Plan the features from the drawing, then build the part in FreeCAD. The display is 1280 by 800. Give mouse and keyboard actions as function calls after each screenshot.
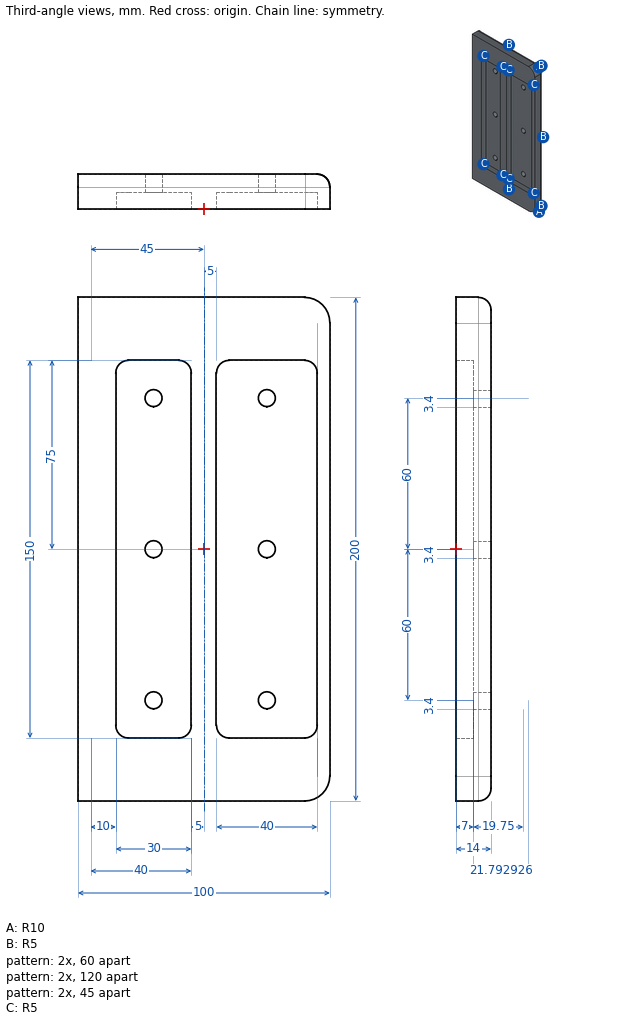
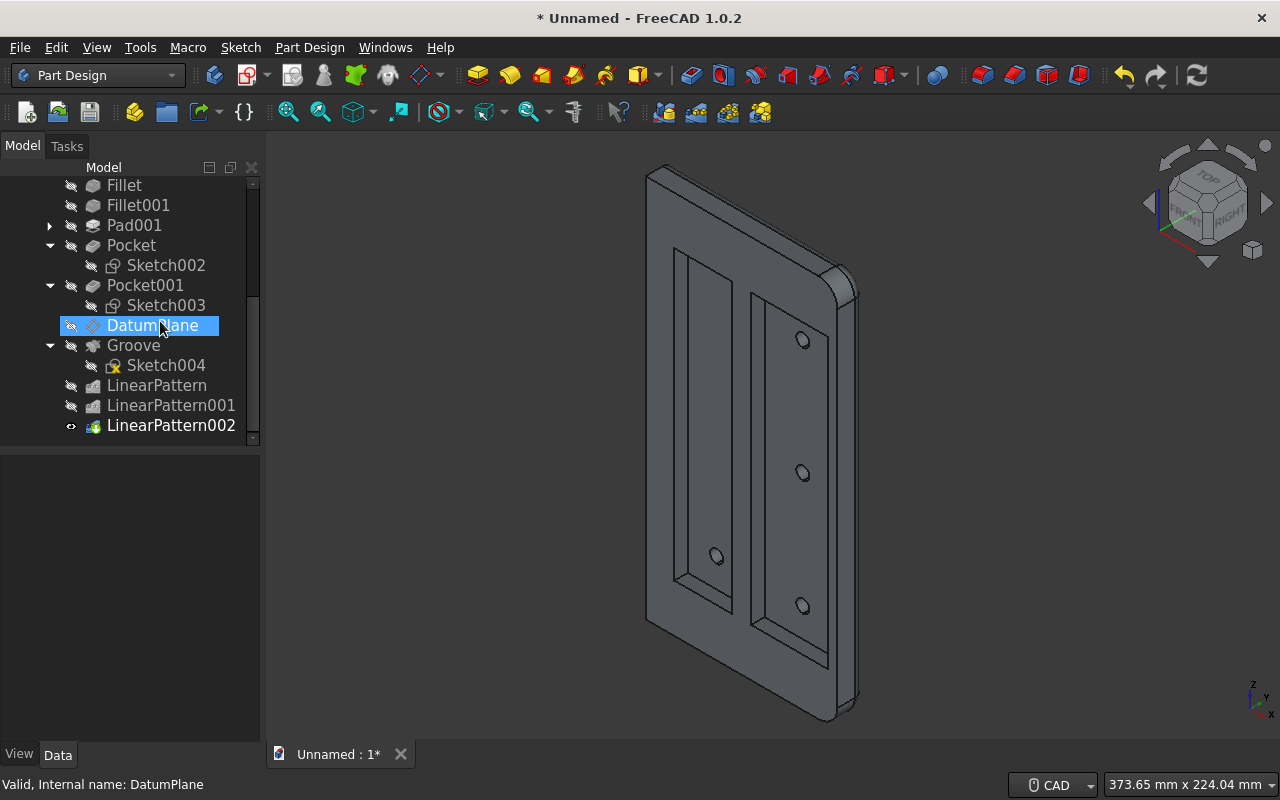
scroll(140, 301, up, 15)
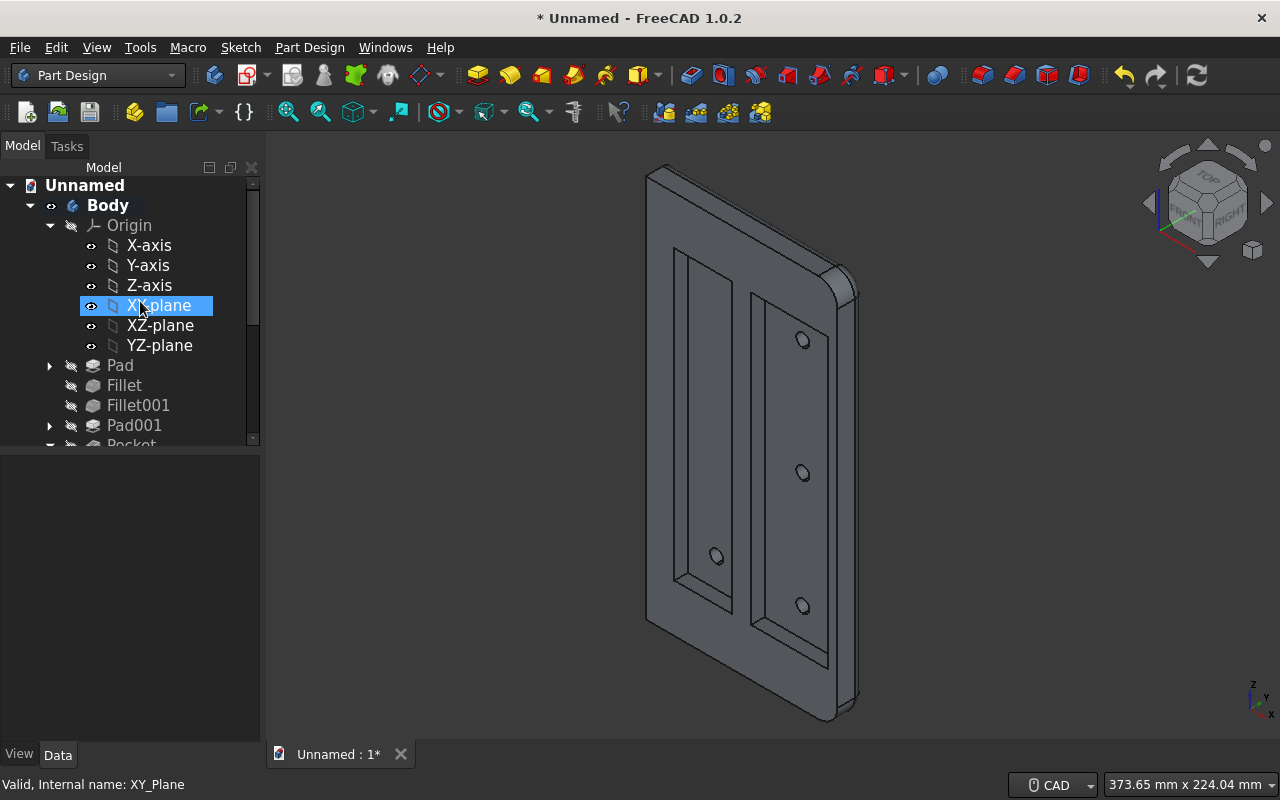
click(136, 346)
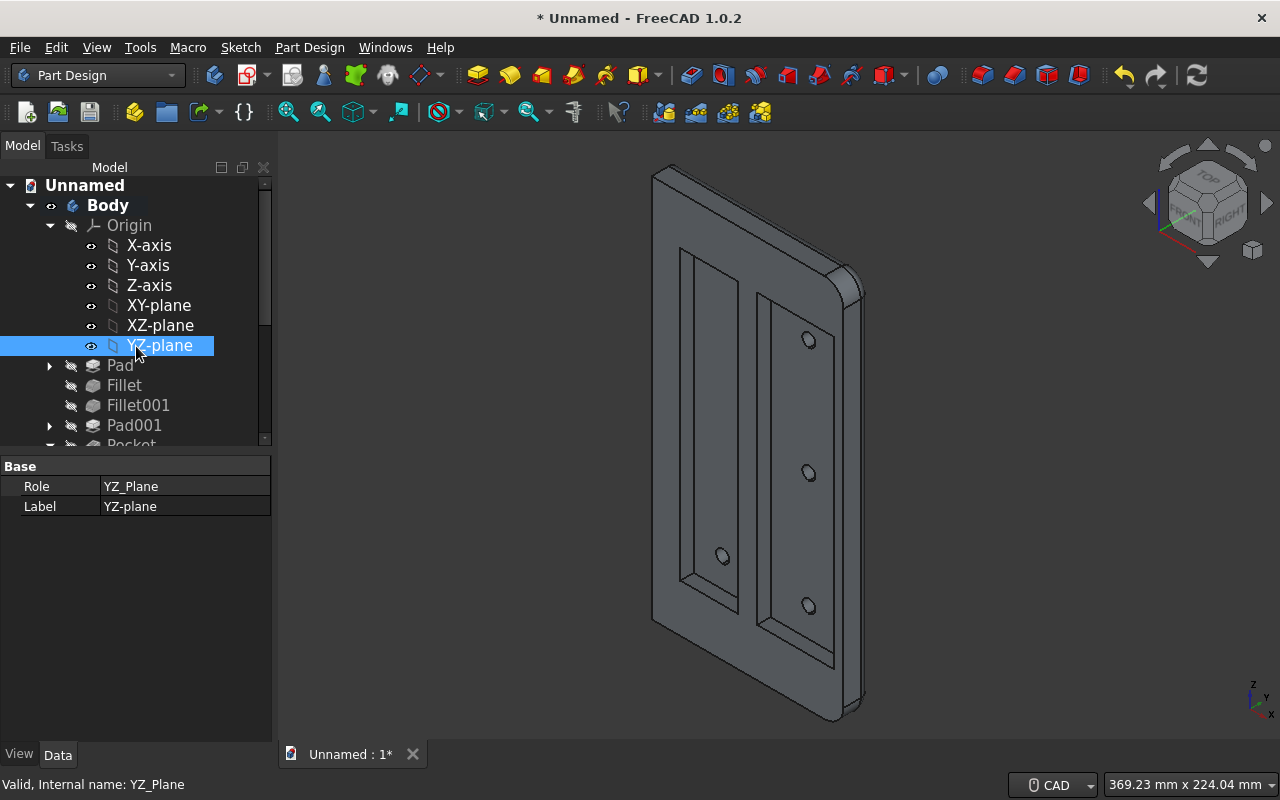
click(420, 76)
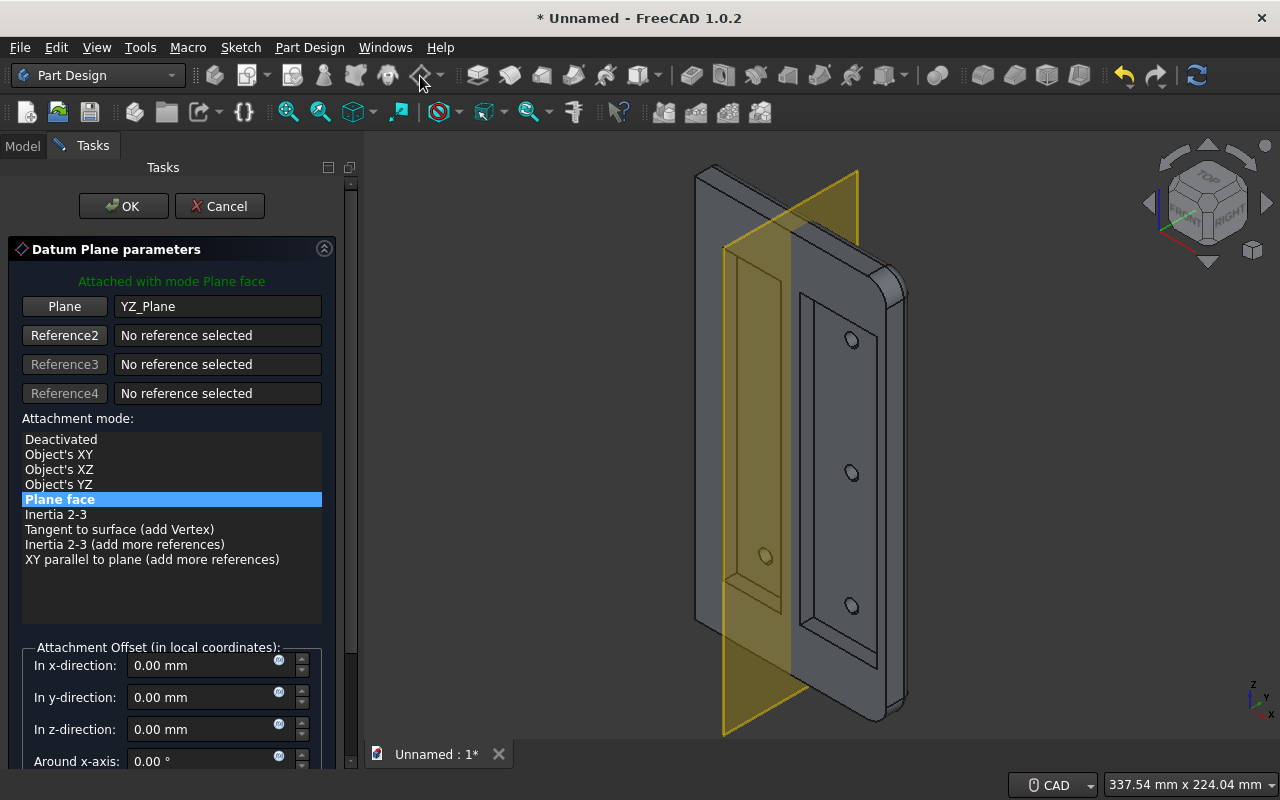
triple_click(210, 729)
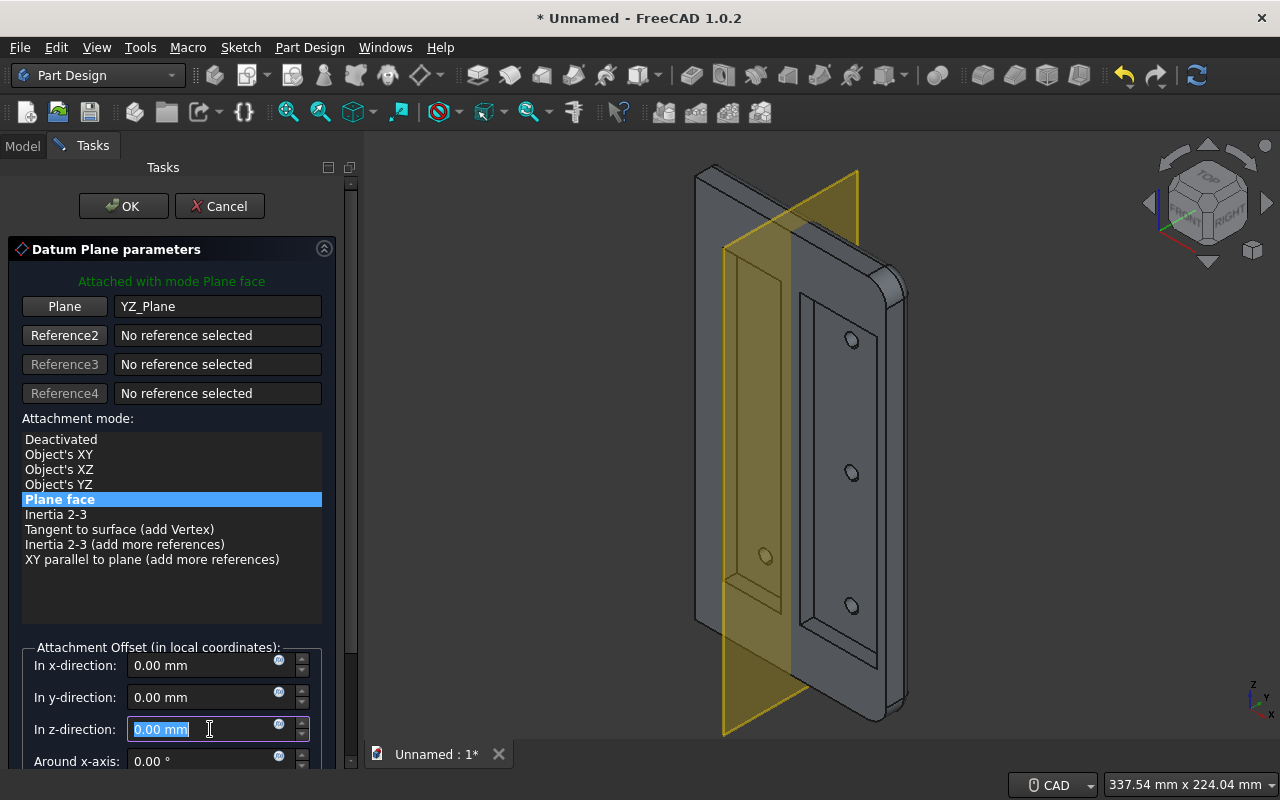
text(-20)
key(Tab)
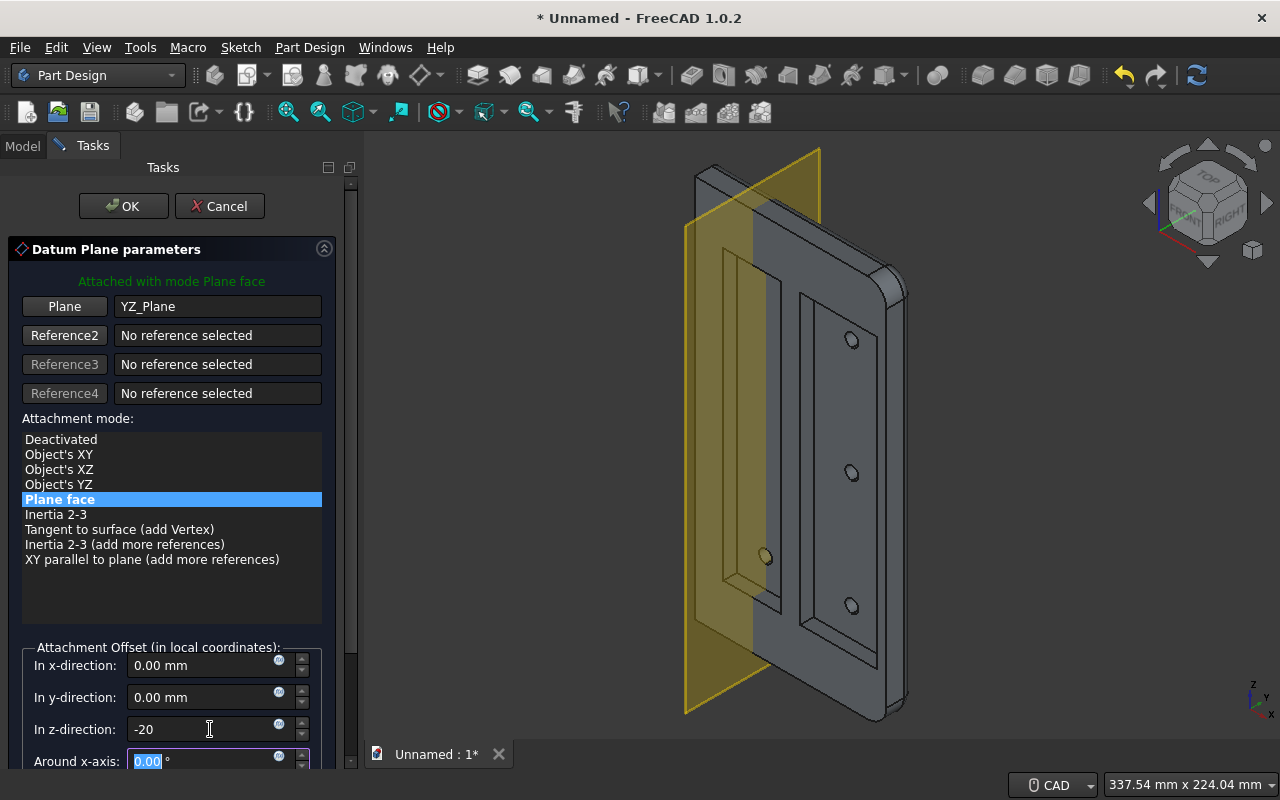
click(124, 206)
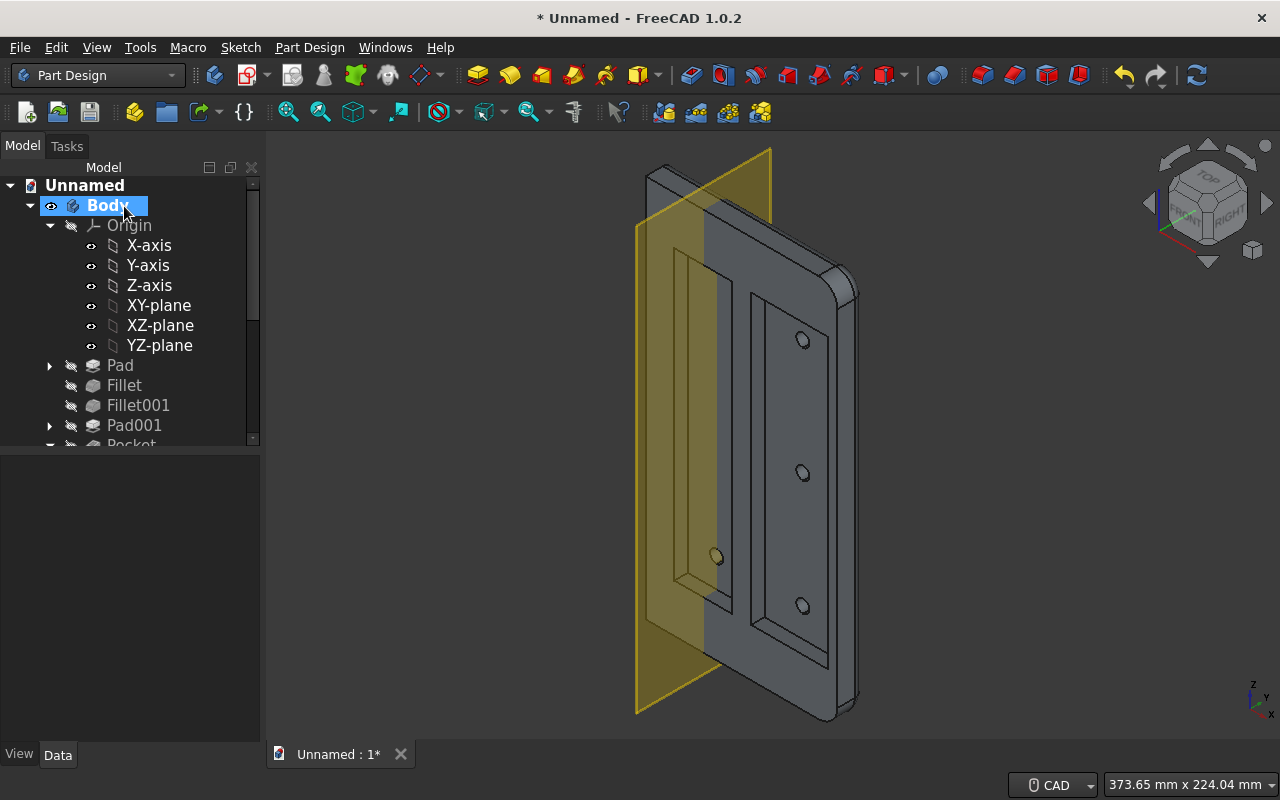
scroll(100, 321, down, 3)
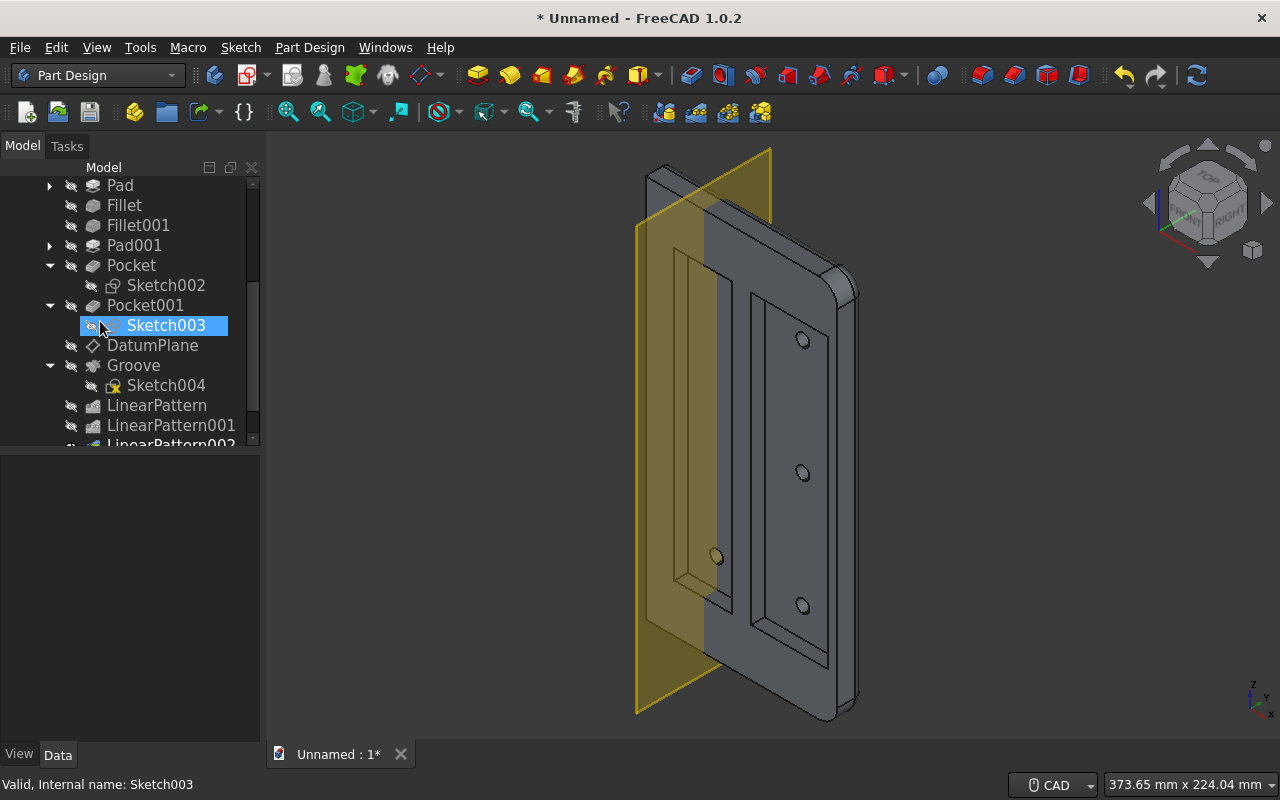
scroll(140, 321, up, 15)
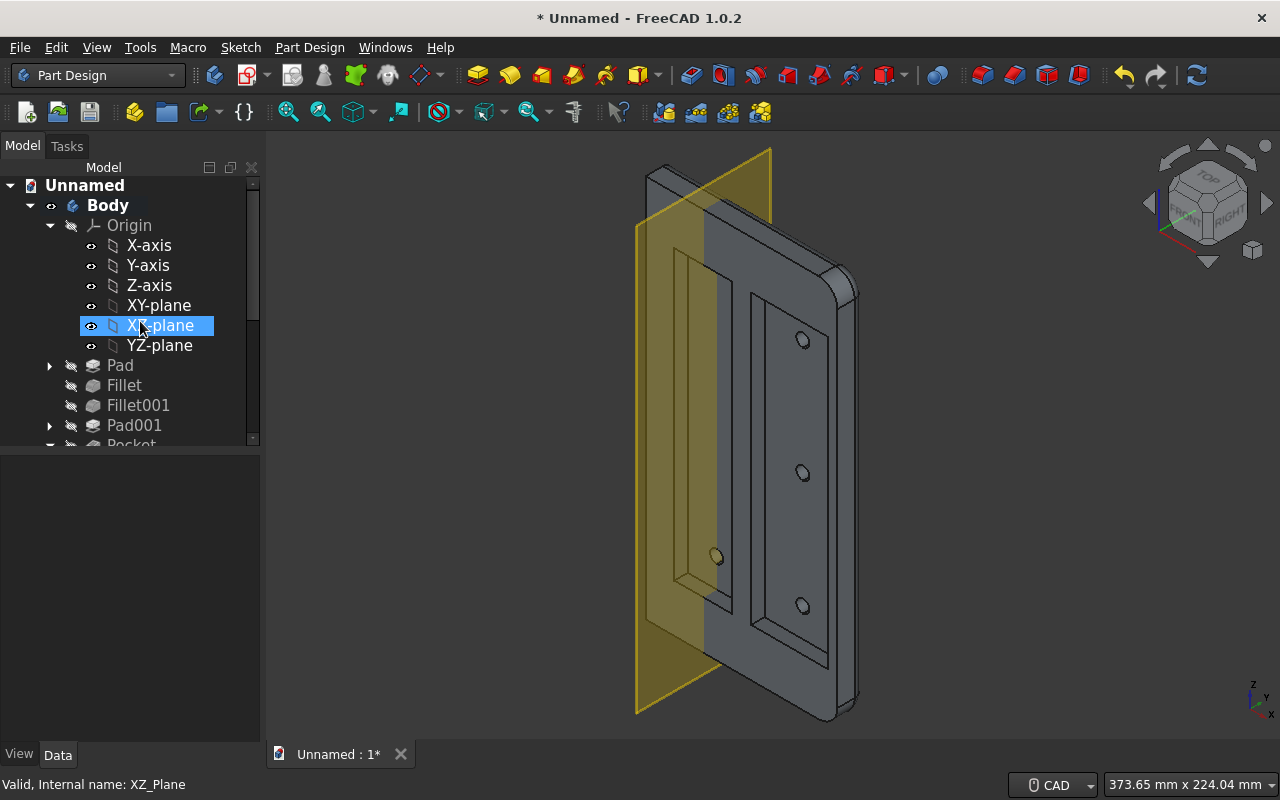
scroll(100, 321, down, 6)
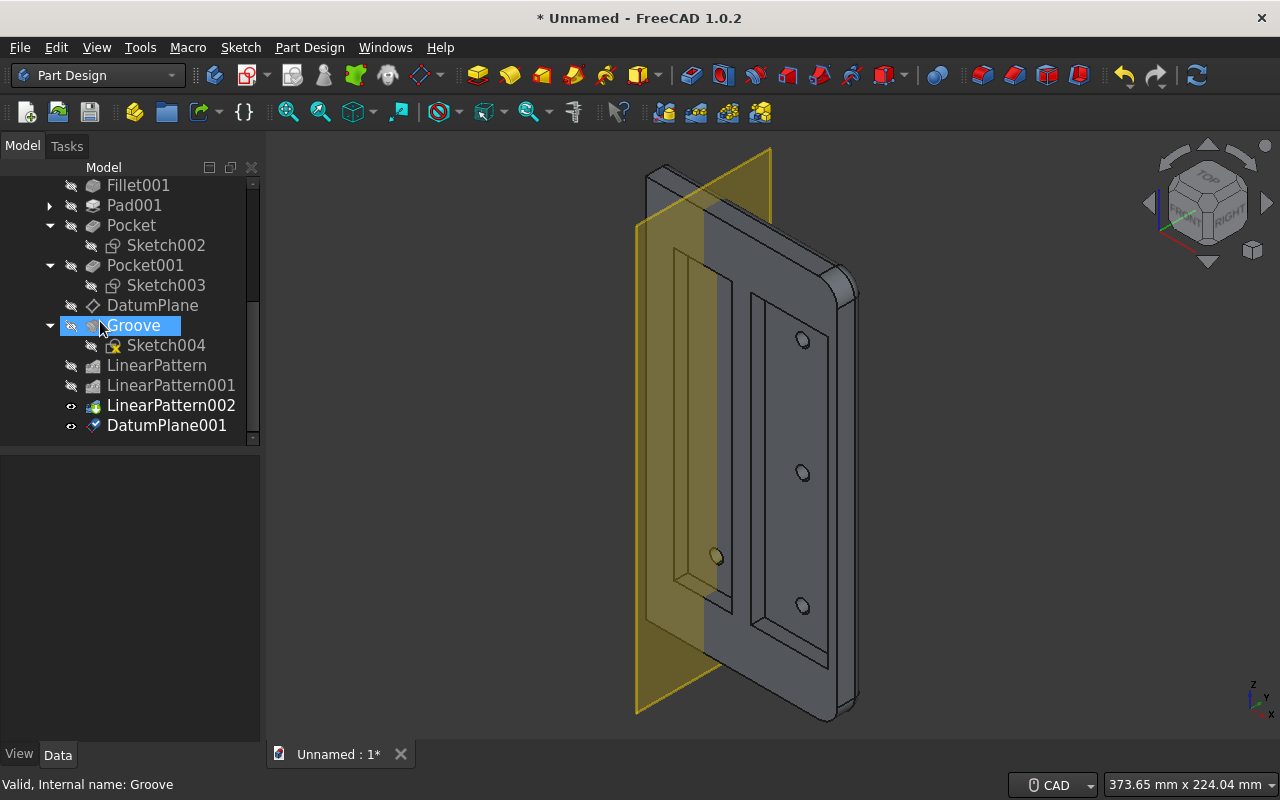
click(116, 426)